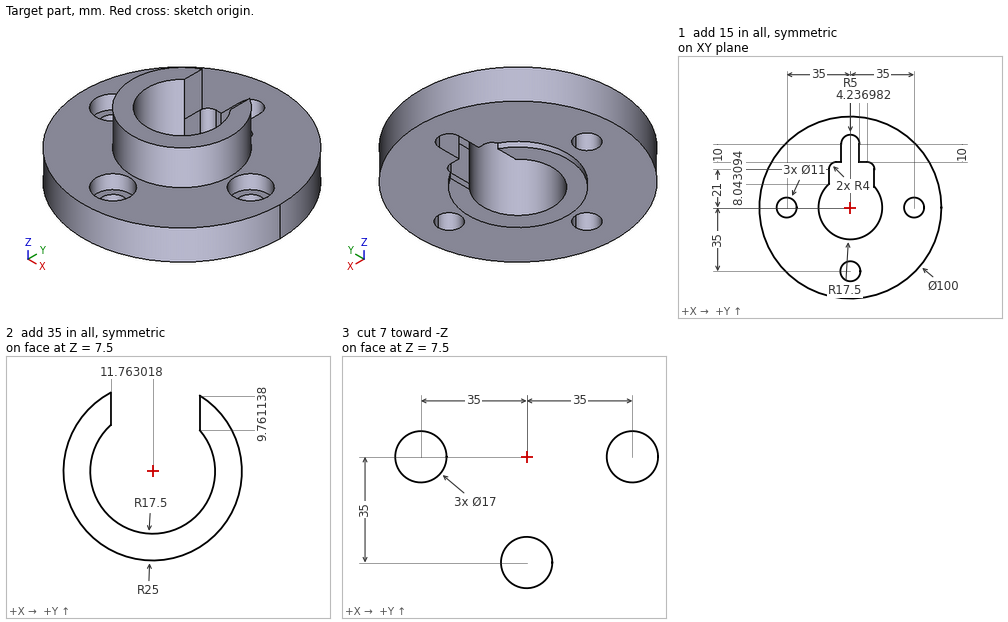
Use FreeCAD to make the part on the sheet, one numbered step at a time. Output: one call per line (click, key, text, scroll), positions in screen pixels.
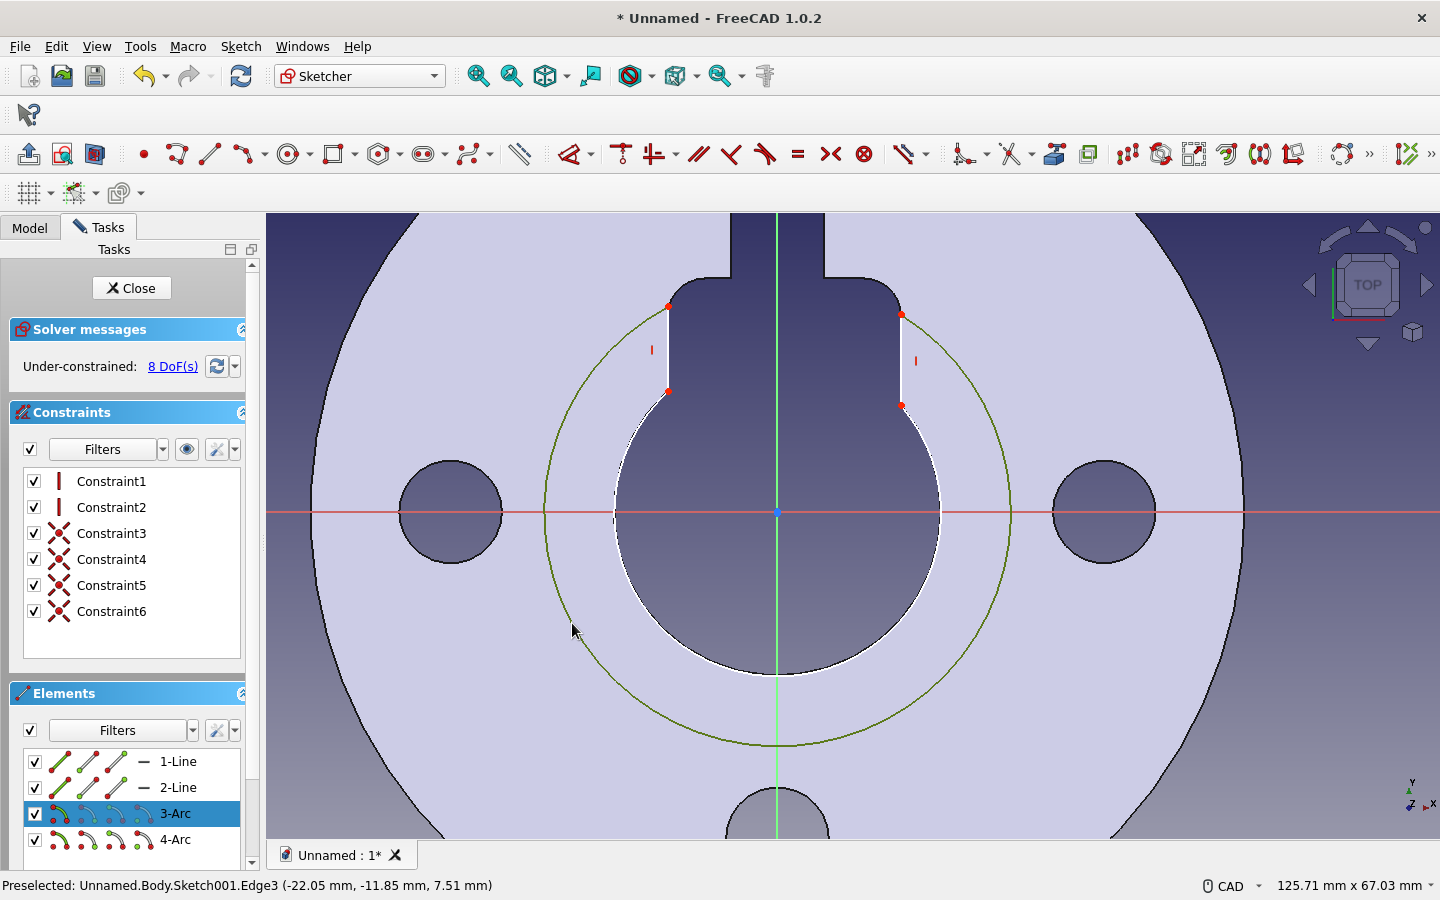
click(640, 602)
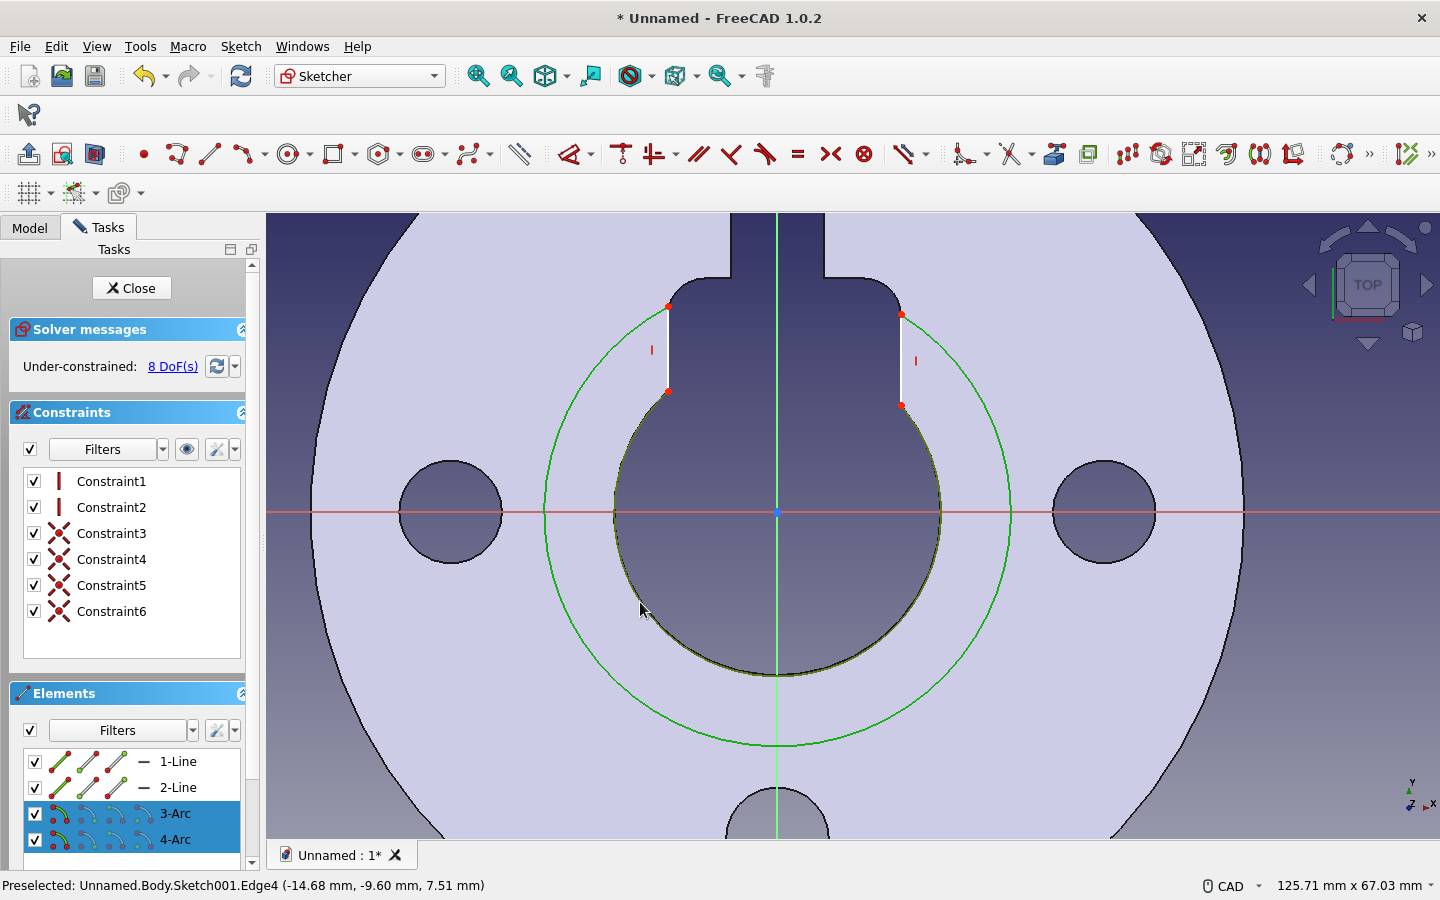
key(c)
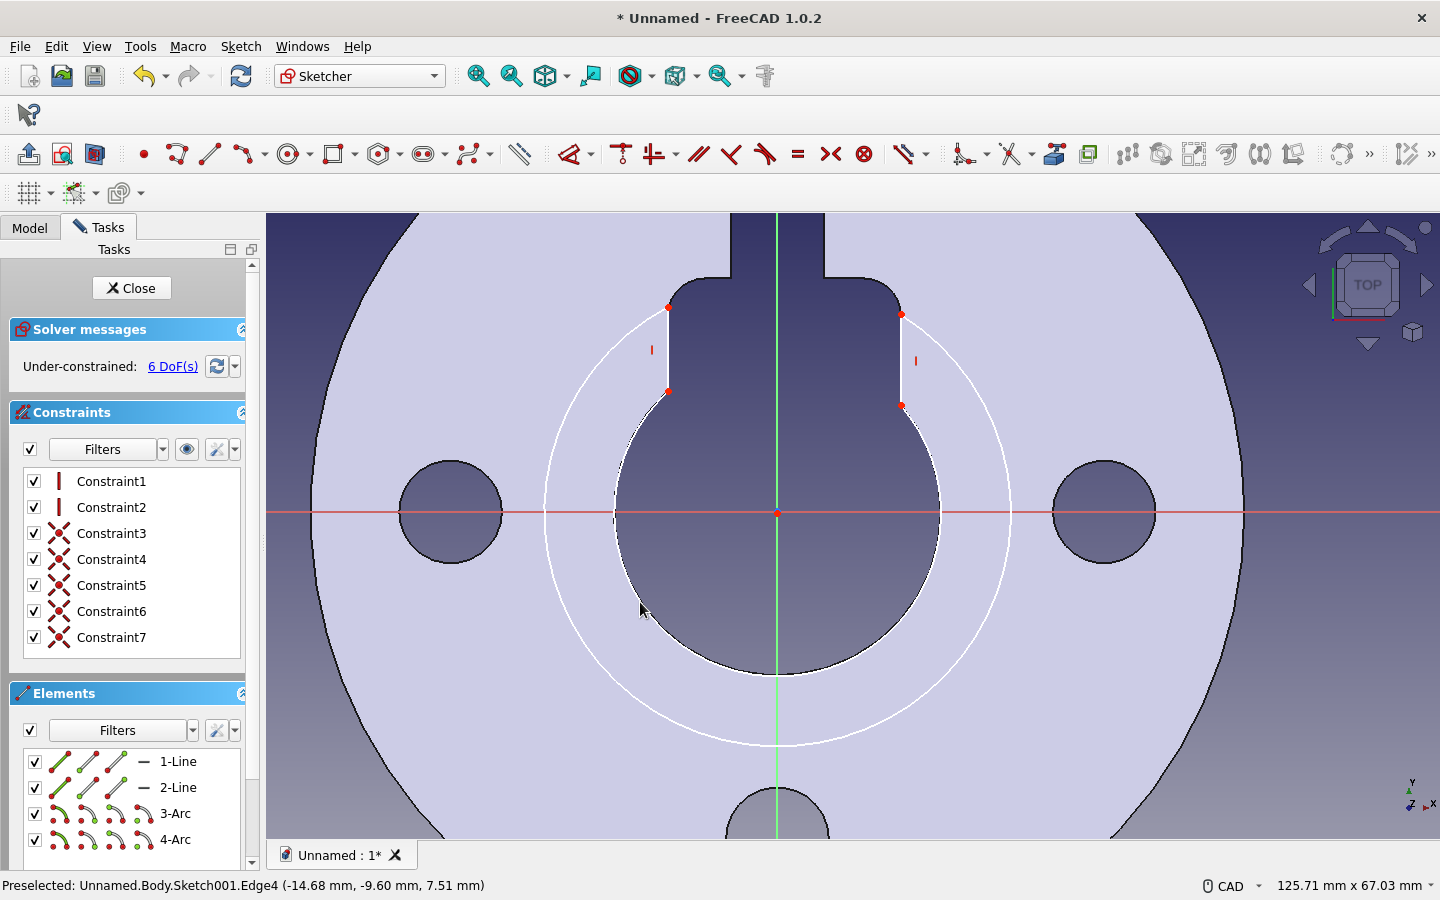
drag(767, 502, 788, 523)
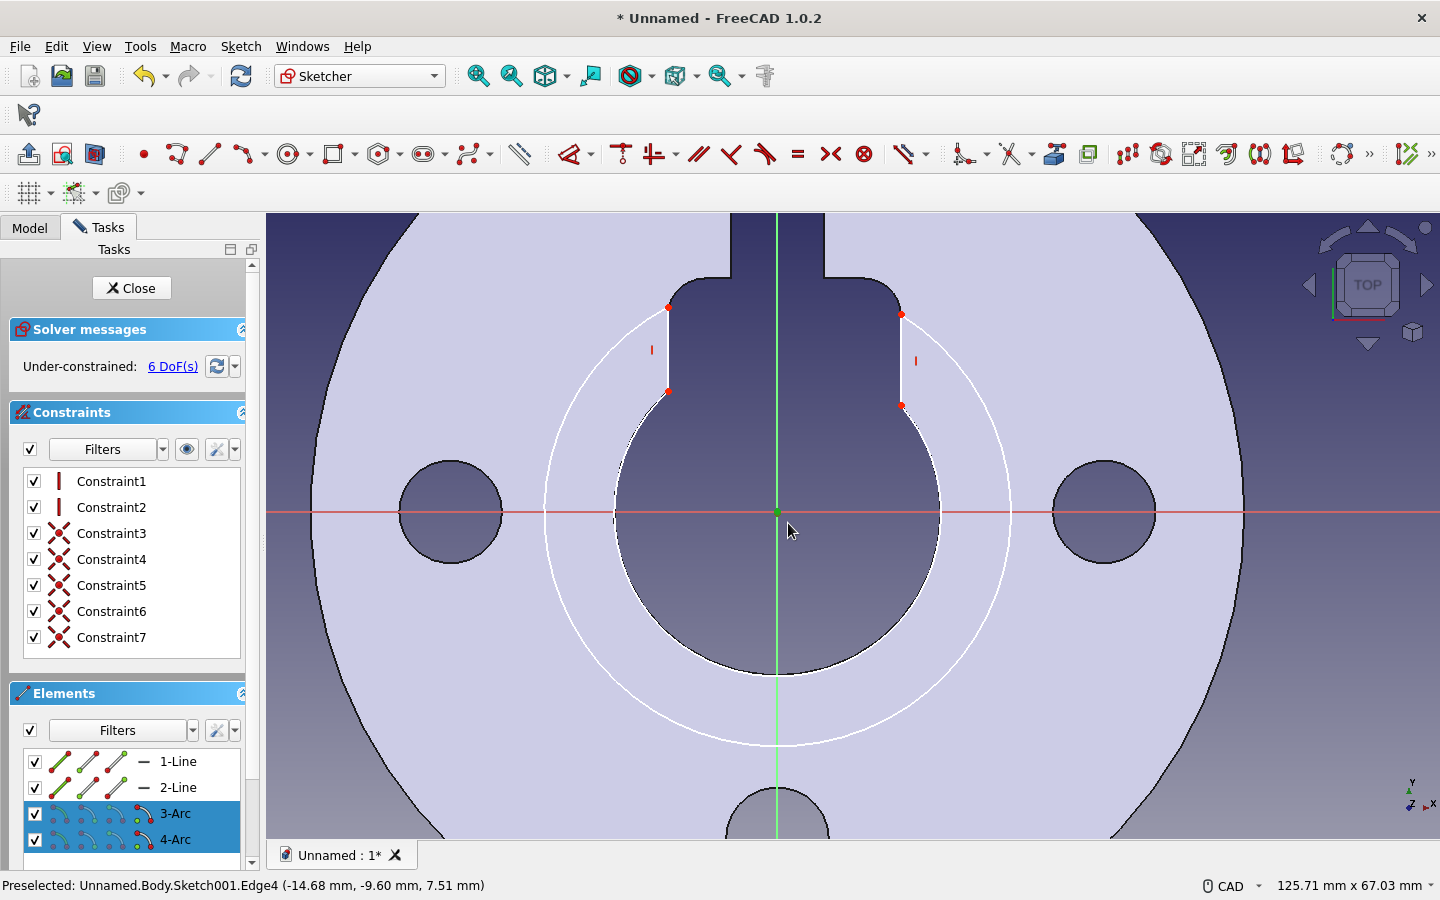
key(c)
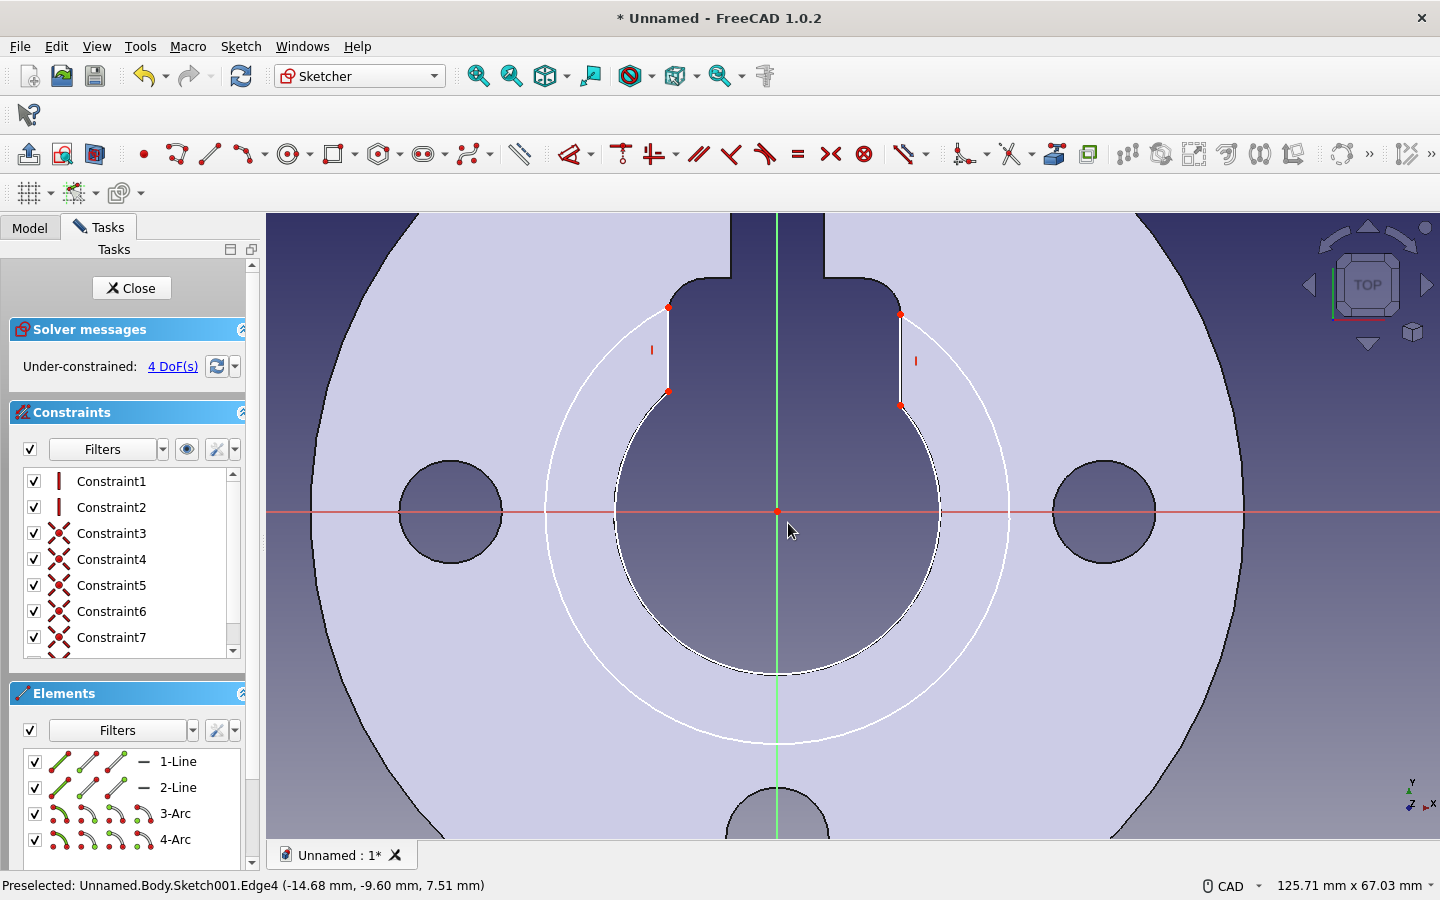
click(568, 154)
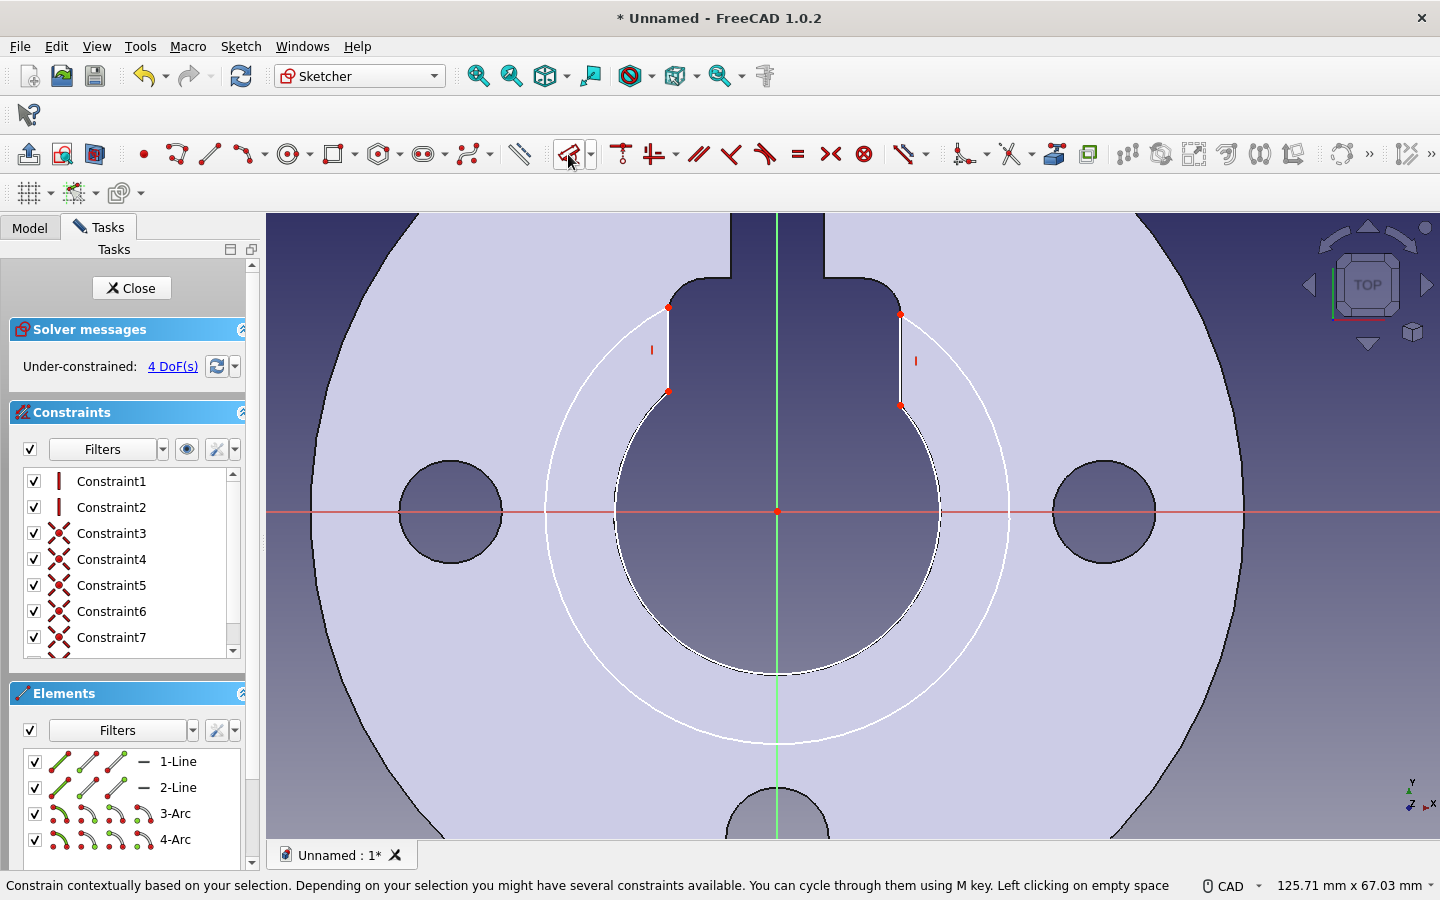
click(573, 621)
click(545, 636)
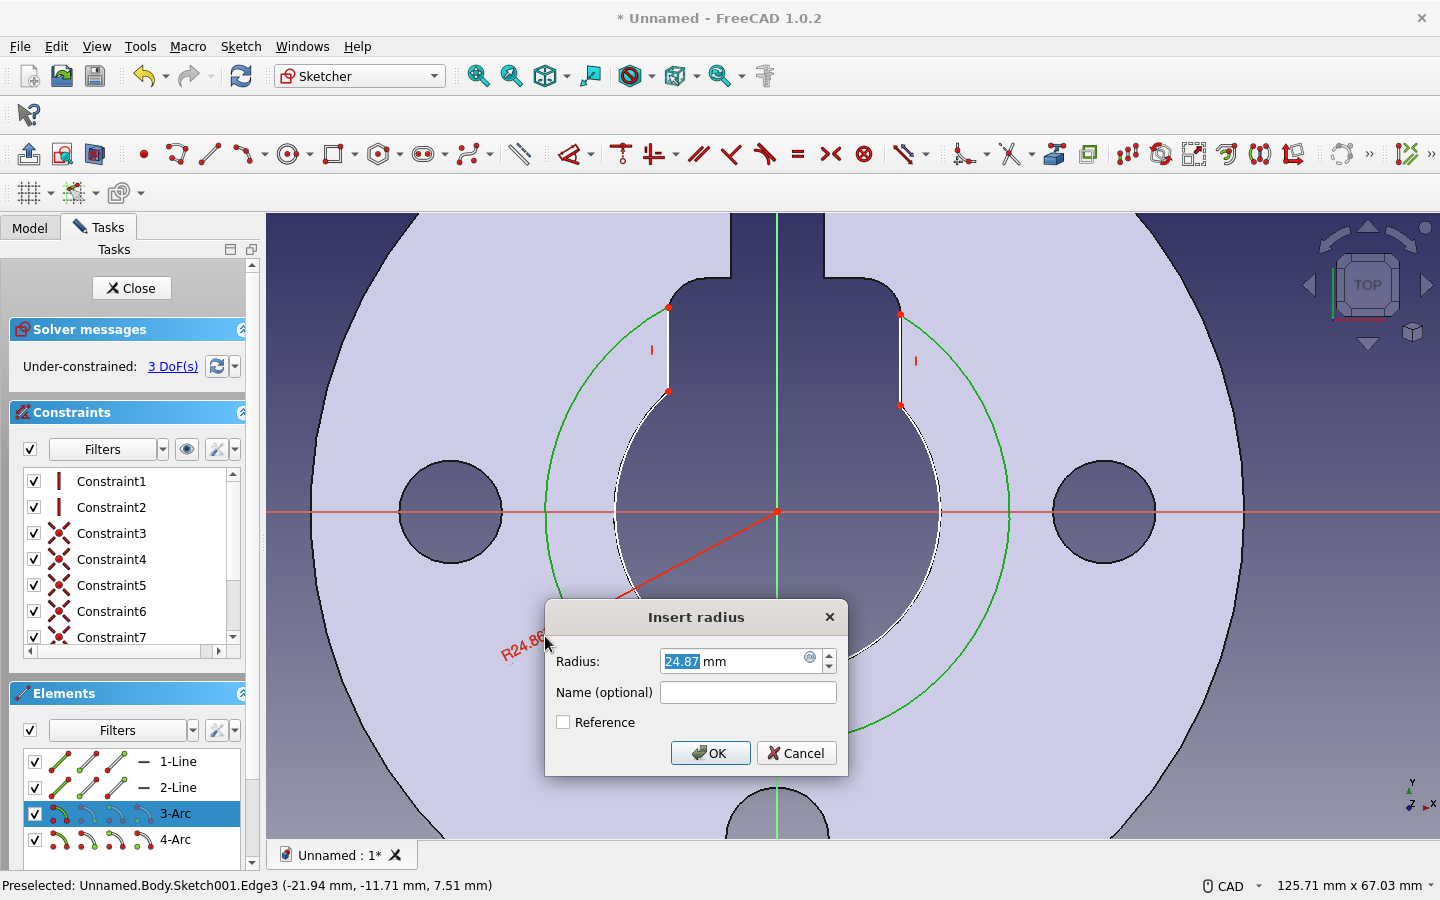
text(25)
key(Return)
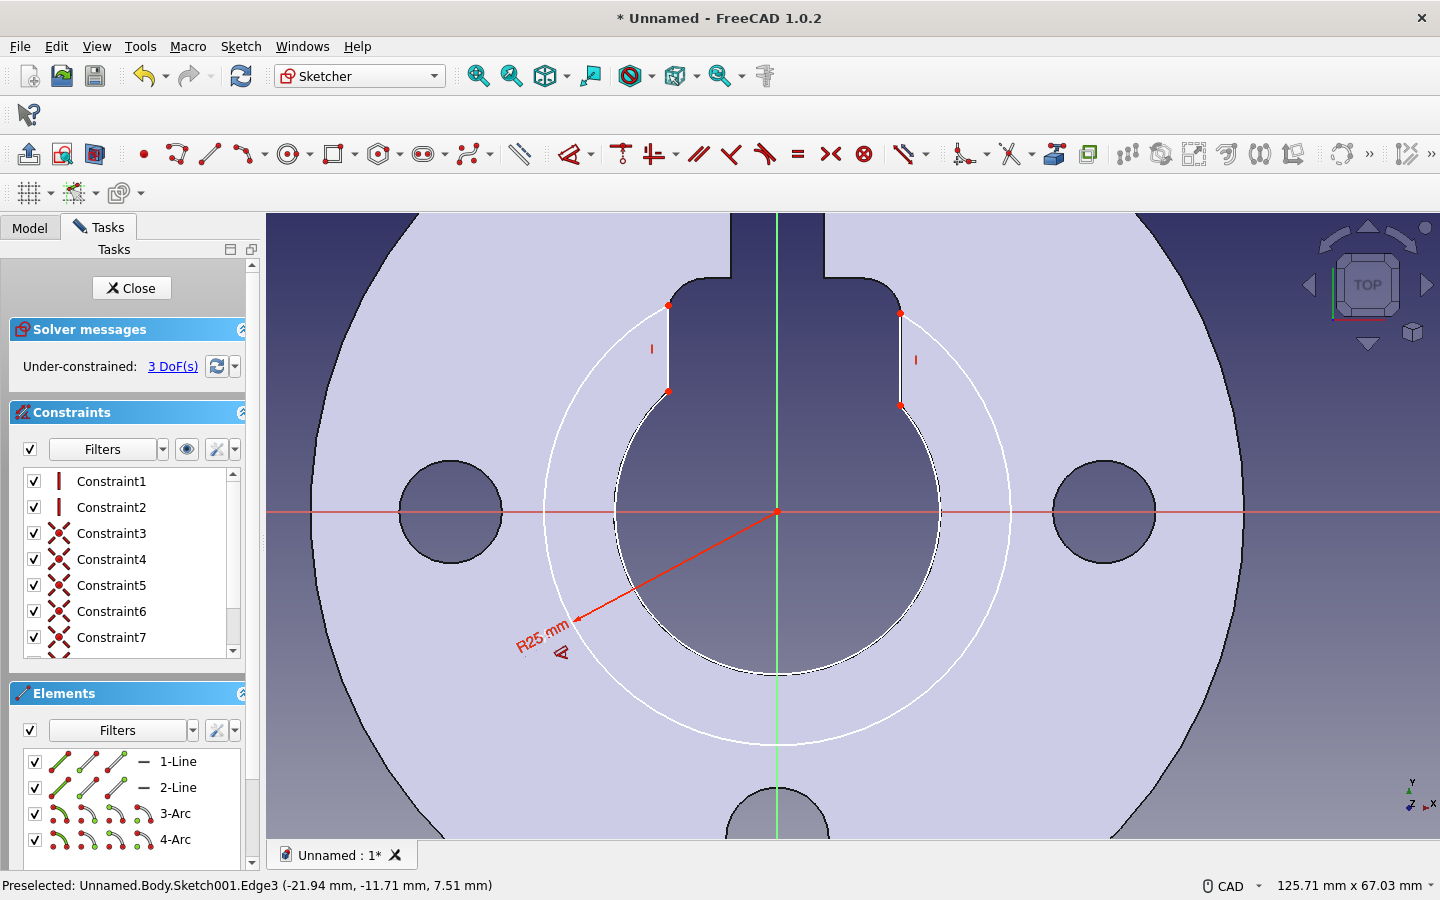
click(641, 600)
click(584, 526)